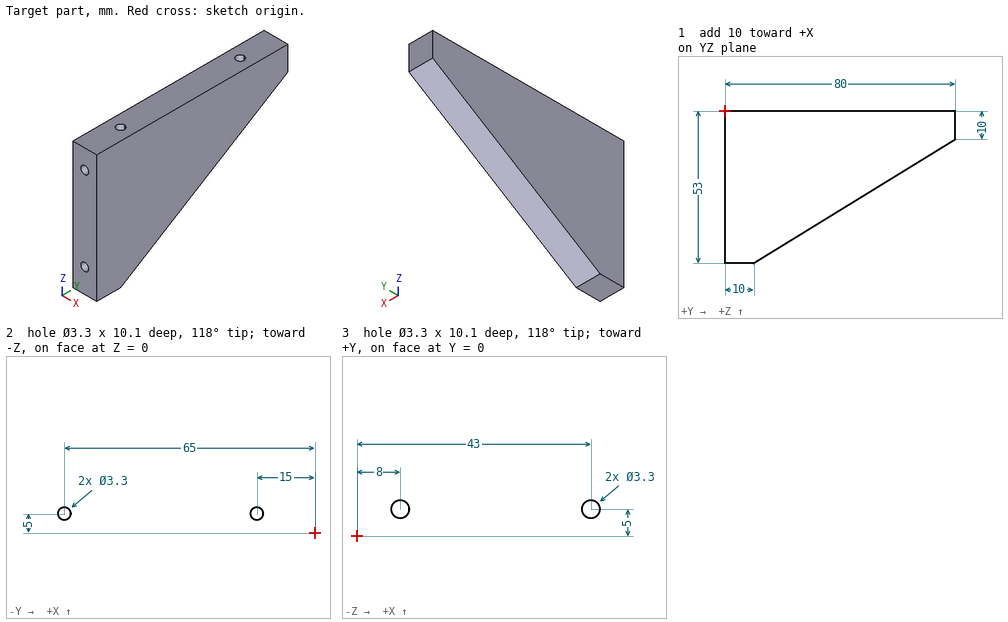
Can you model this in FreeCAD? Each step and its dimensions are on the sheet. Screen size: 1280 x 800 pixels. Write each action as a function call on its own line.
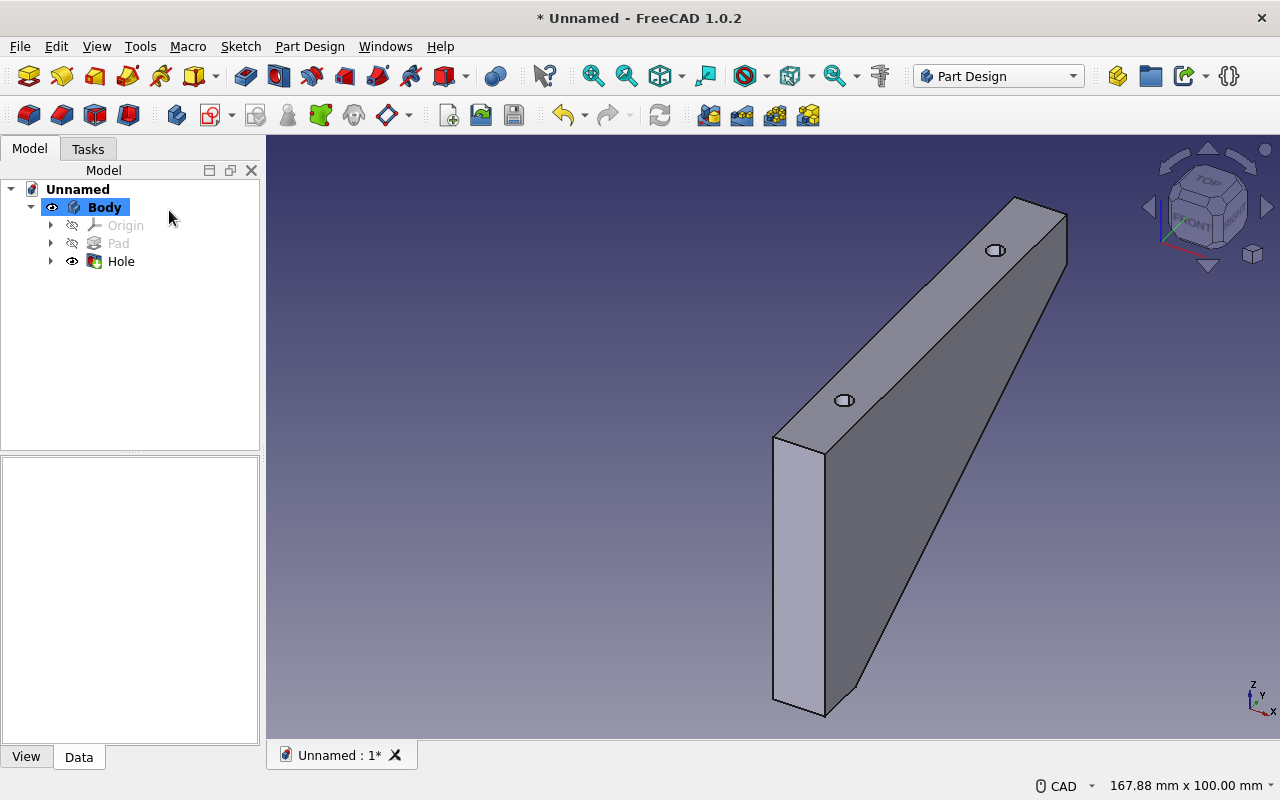
click(799, 651)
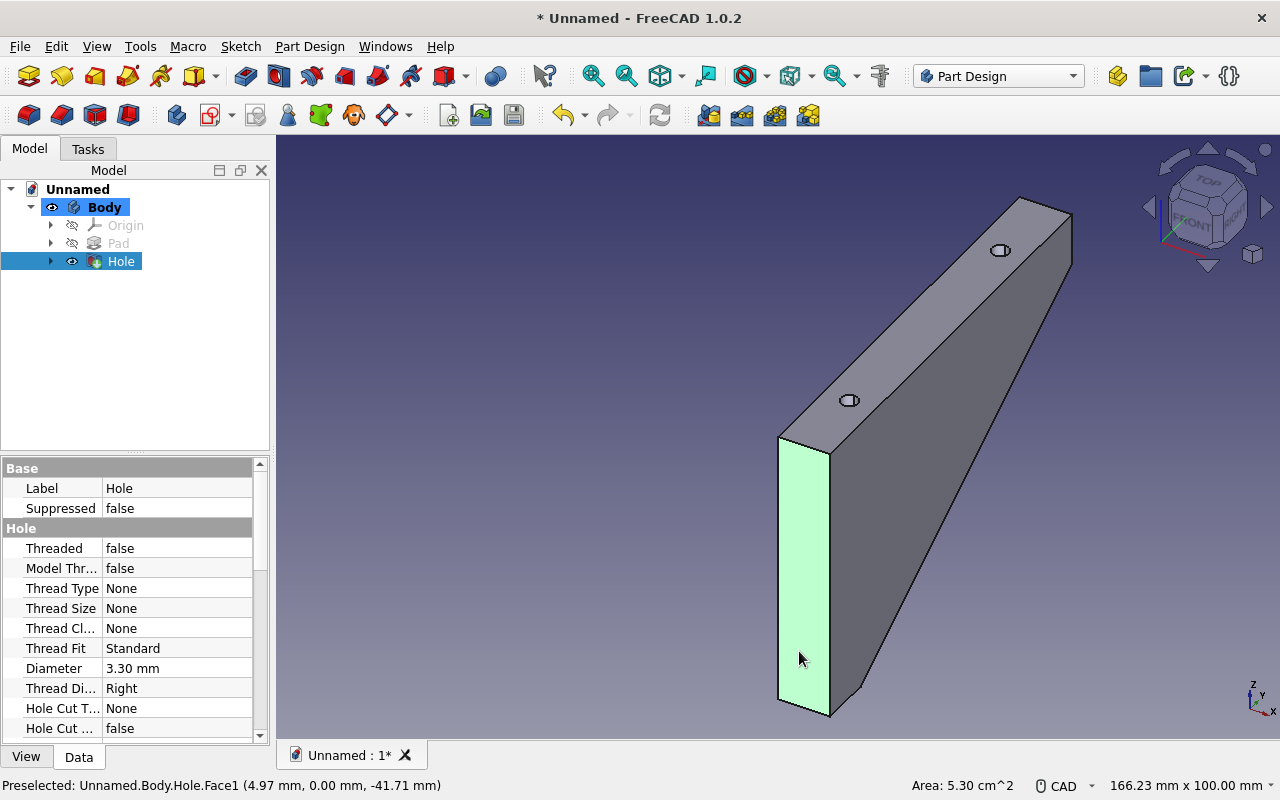
click(210, 116)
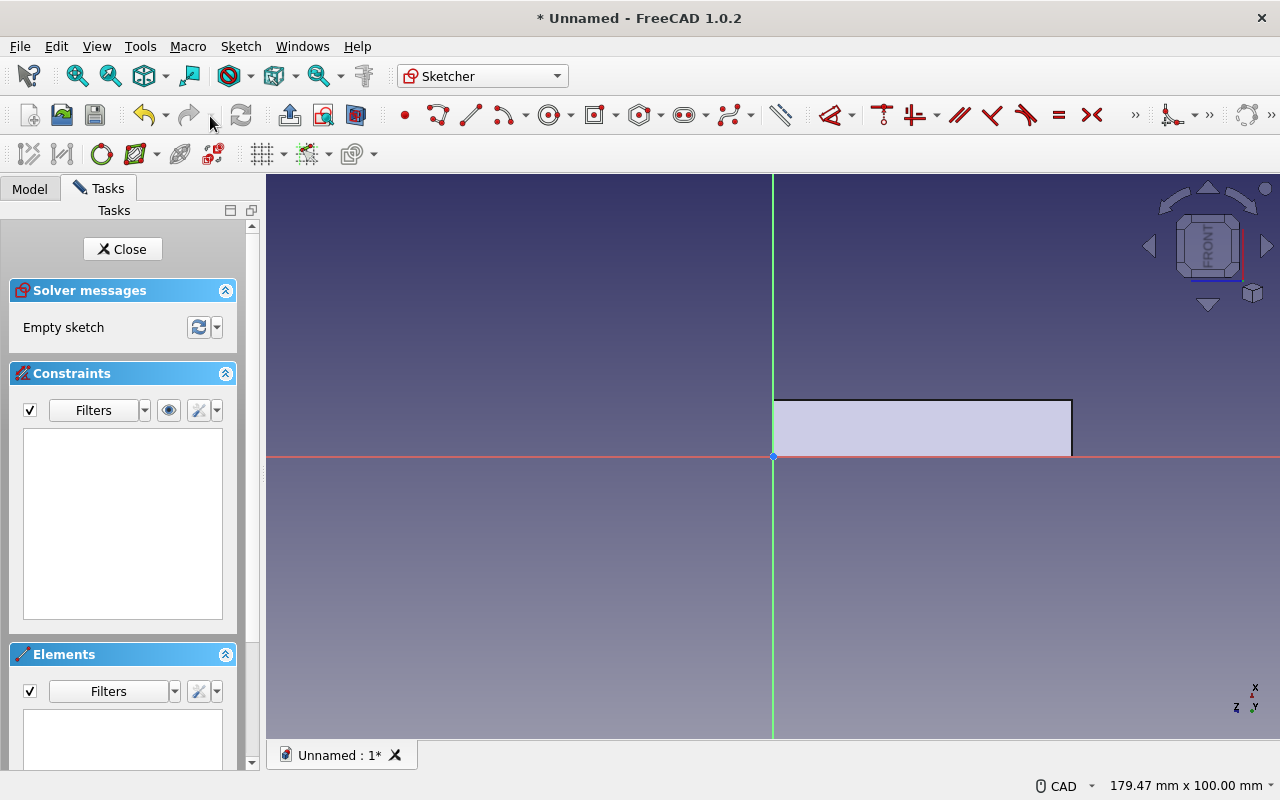
scroll(1058, 422, up, 4)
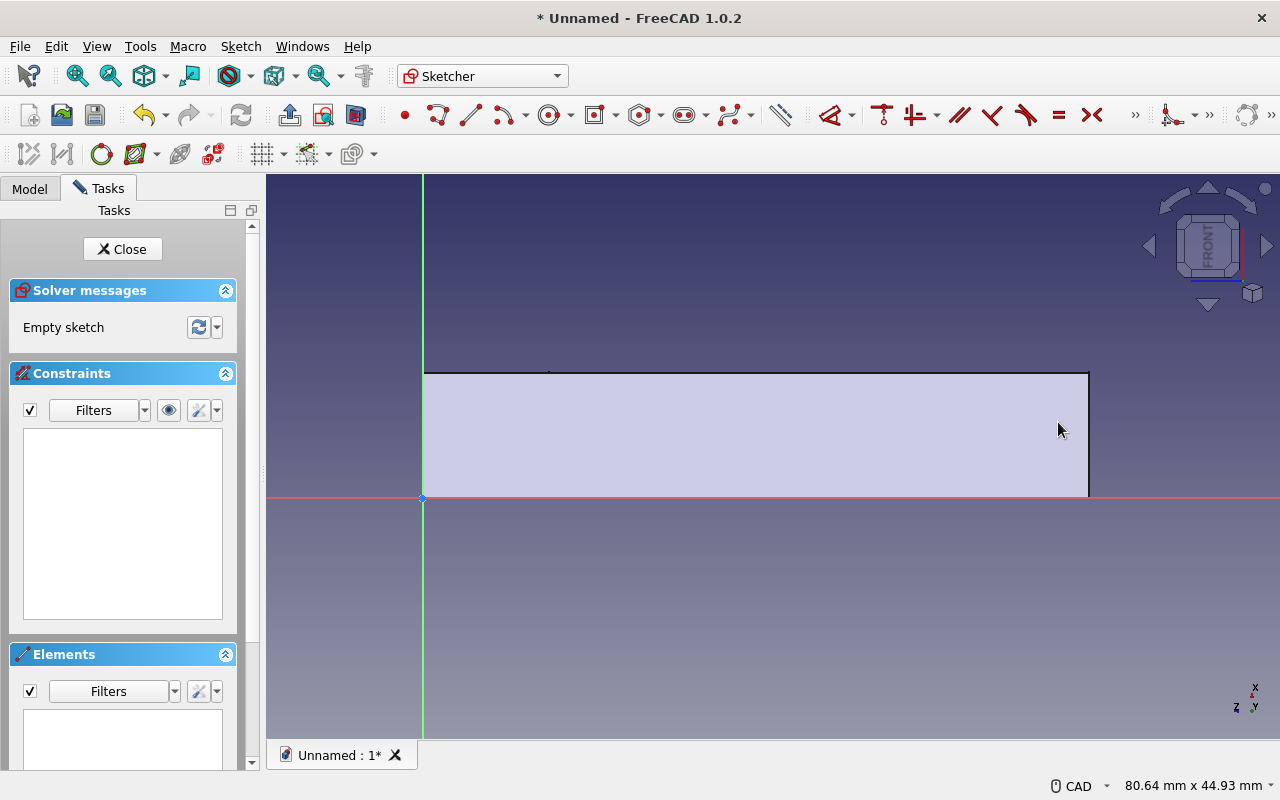
click(548, 116)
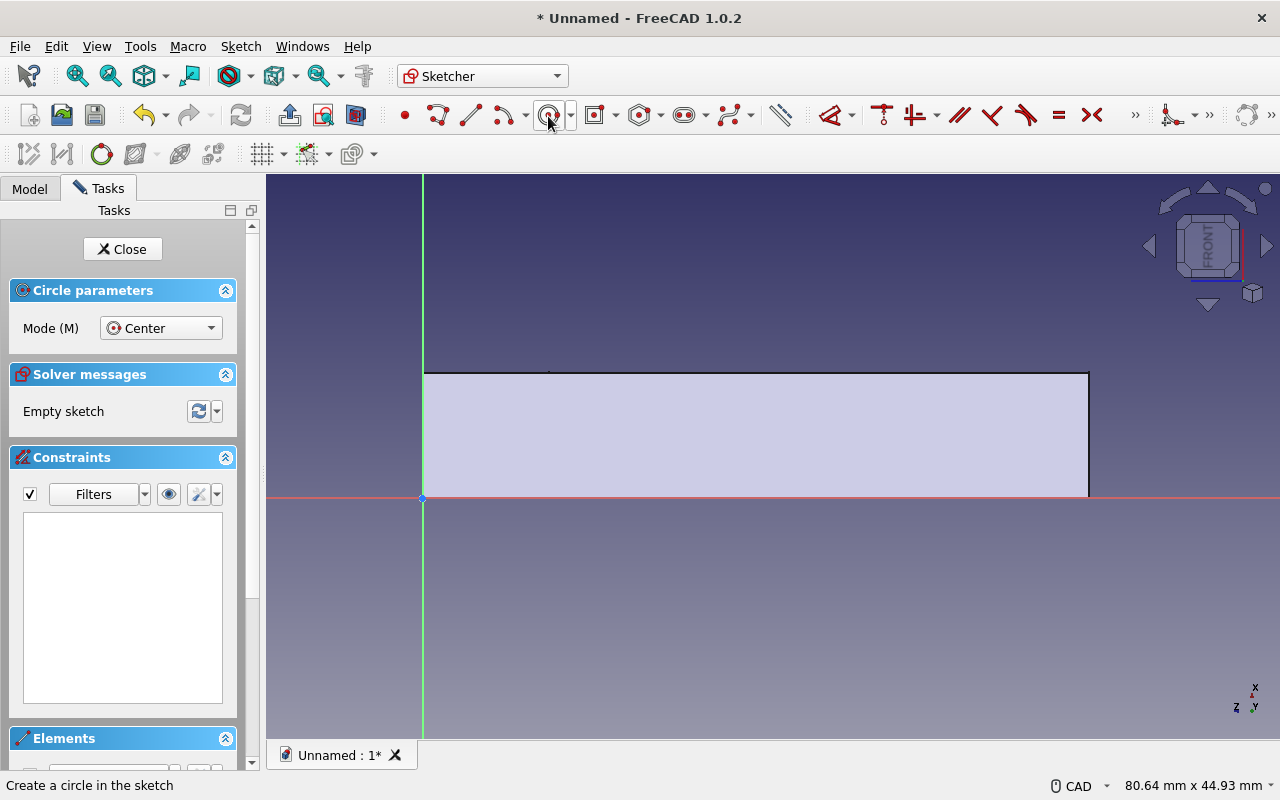
click(963, 435)
move(978, 421)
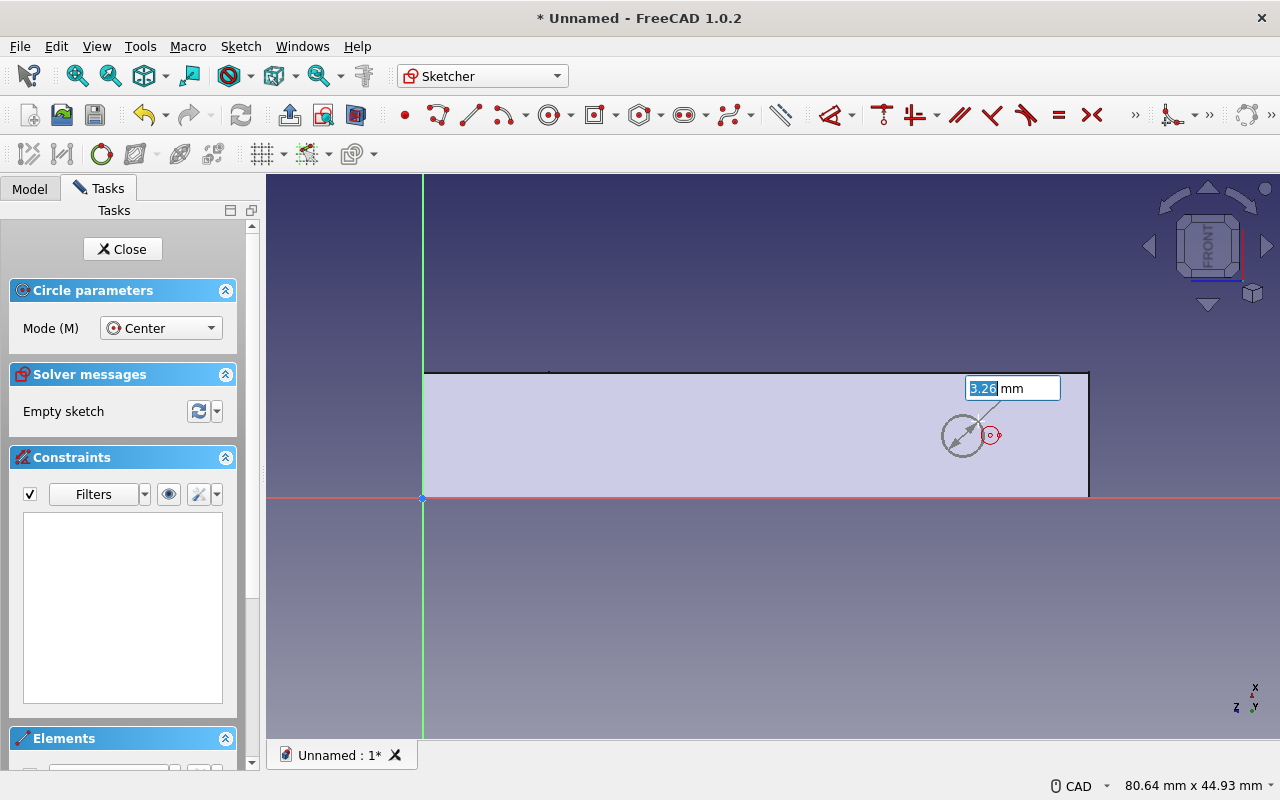
text(3.3)
key(Return)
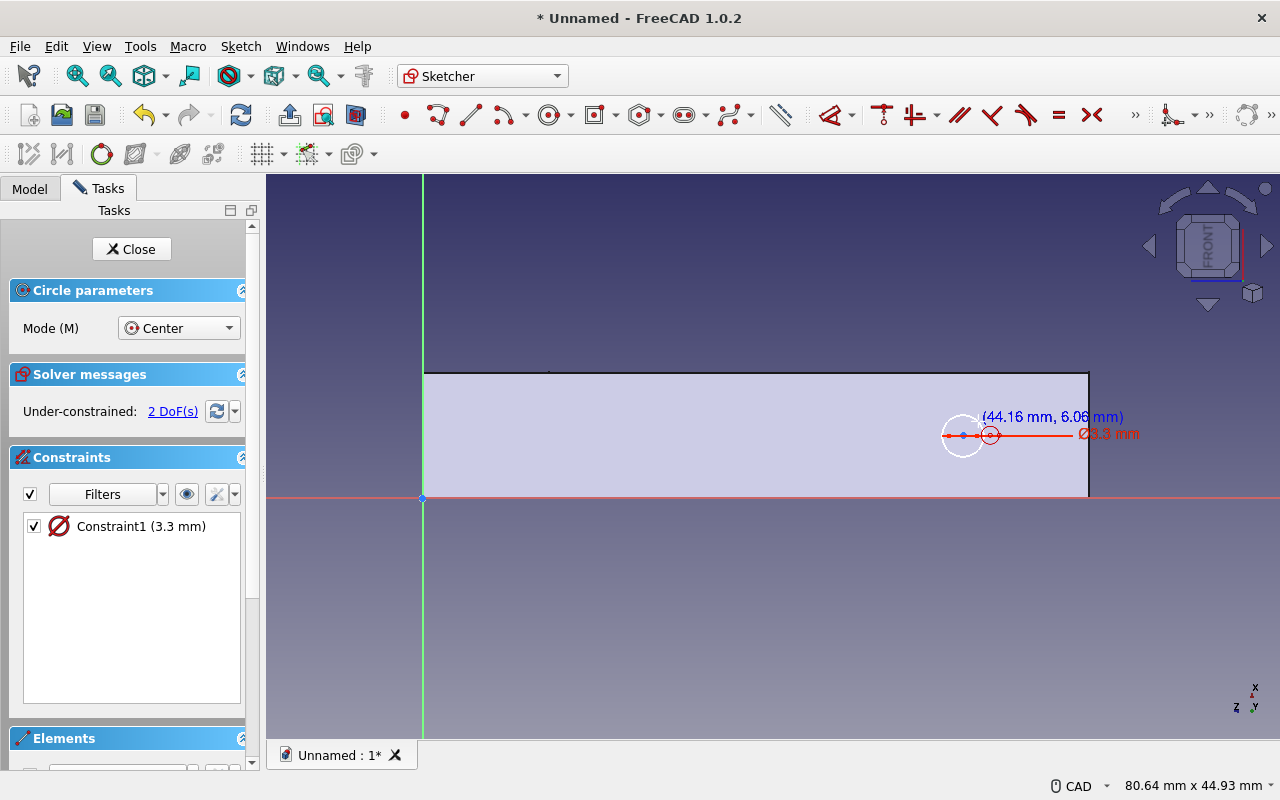
click(523, 435)
move(538, 421)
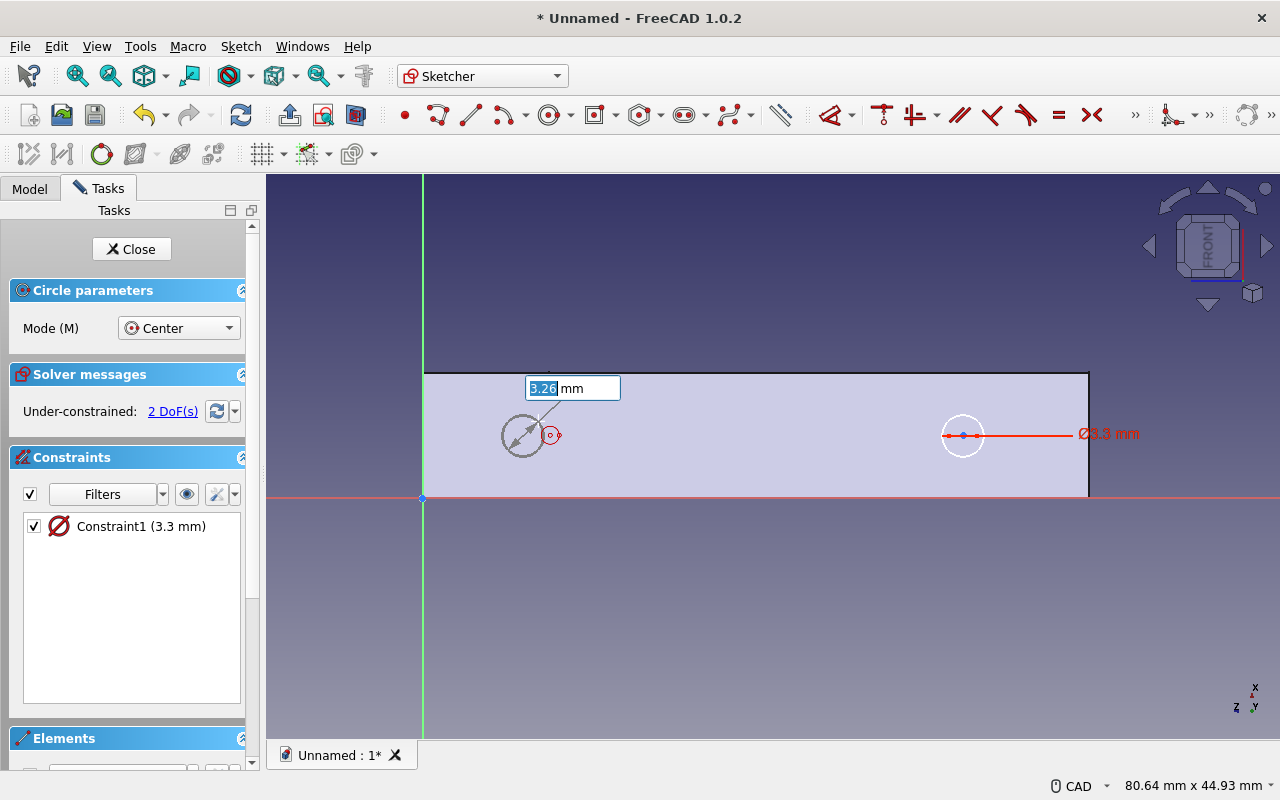
text(3.3)
key(Return)
key(Escape)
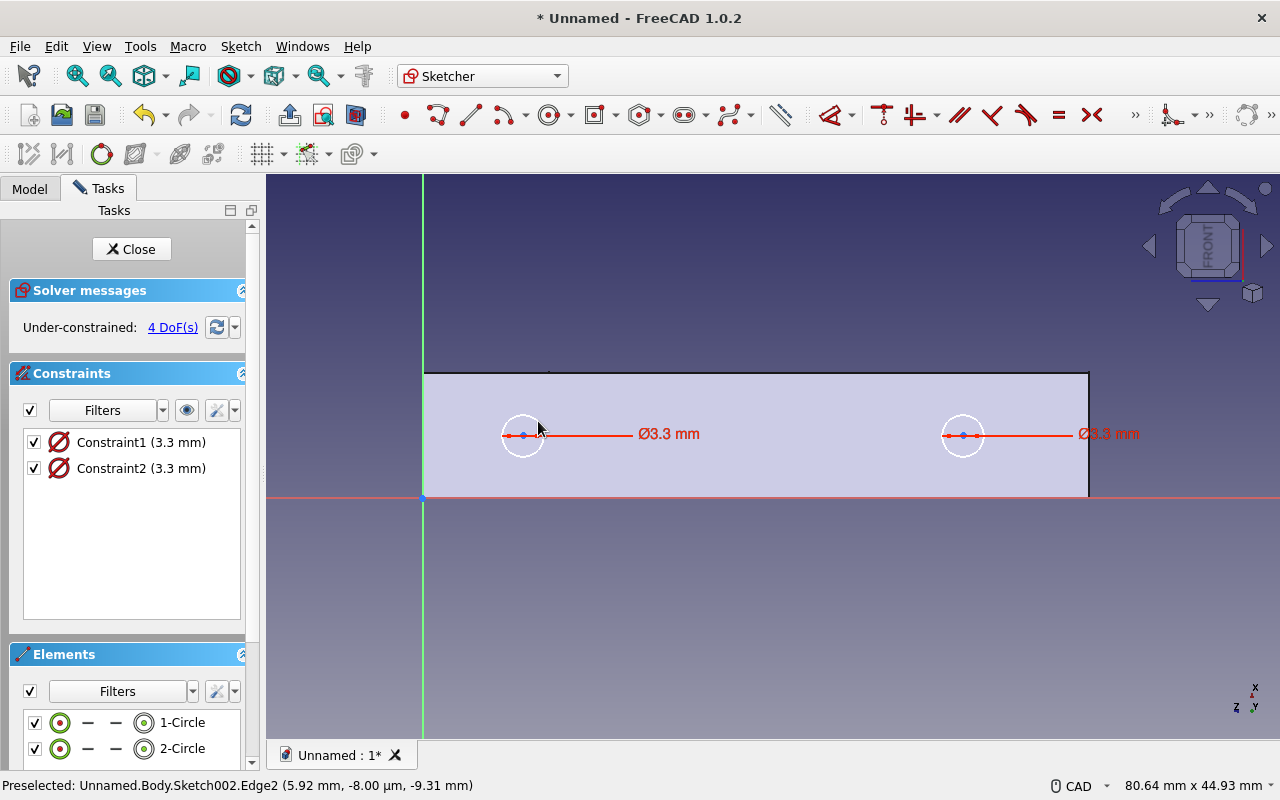
click(963, 436)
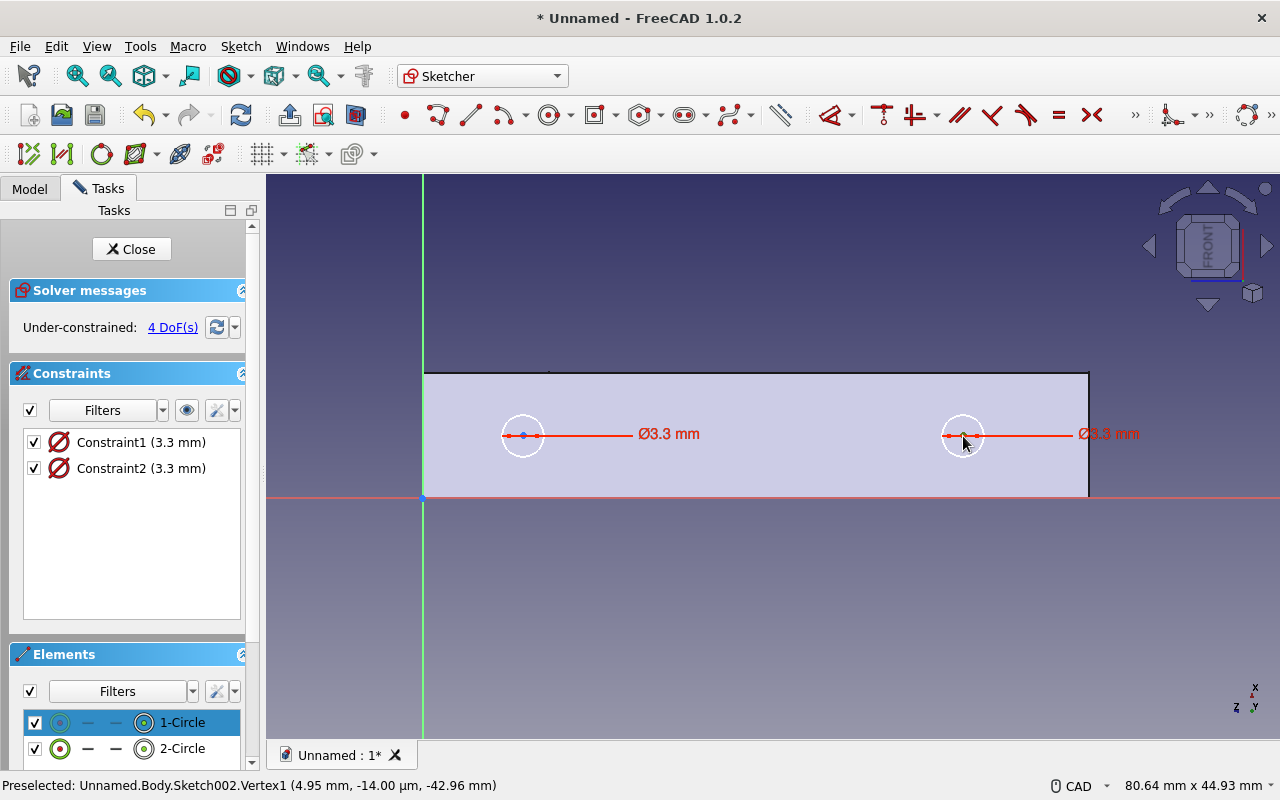
click(523, 436)